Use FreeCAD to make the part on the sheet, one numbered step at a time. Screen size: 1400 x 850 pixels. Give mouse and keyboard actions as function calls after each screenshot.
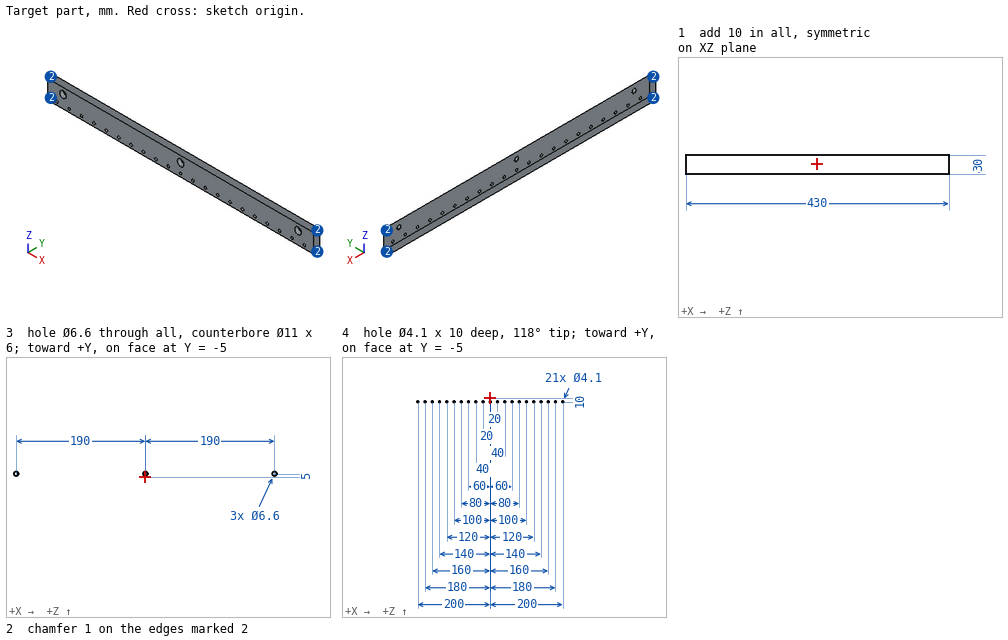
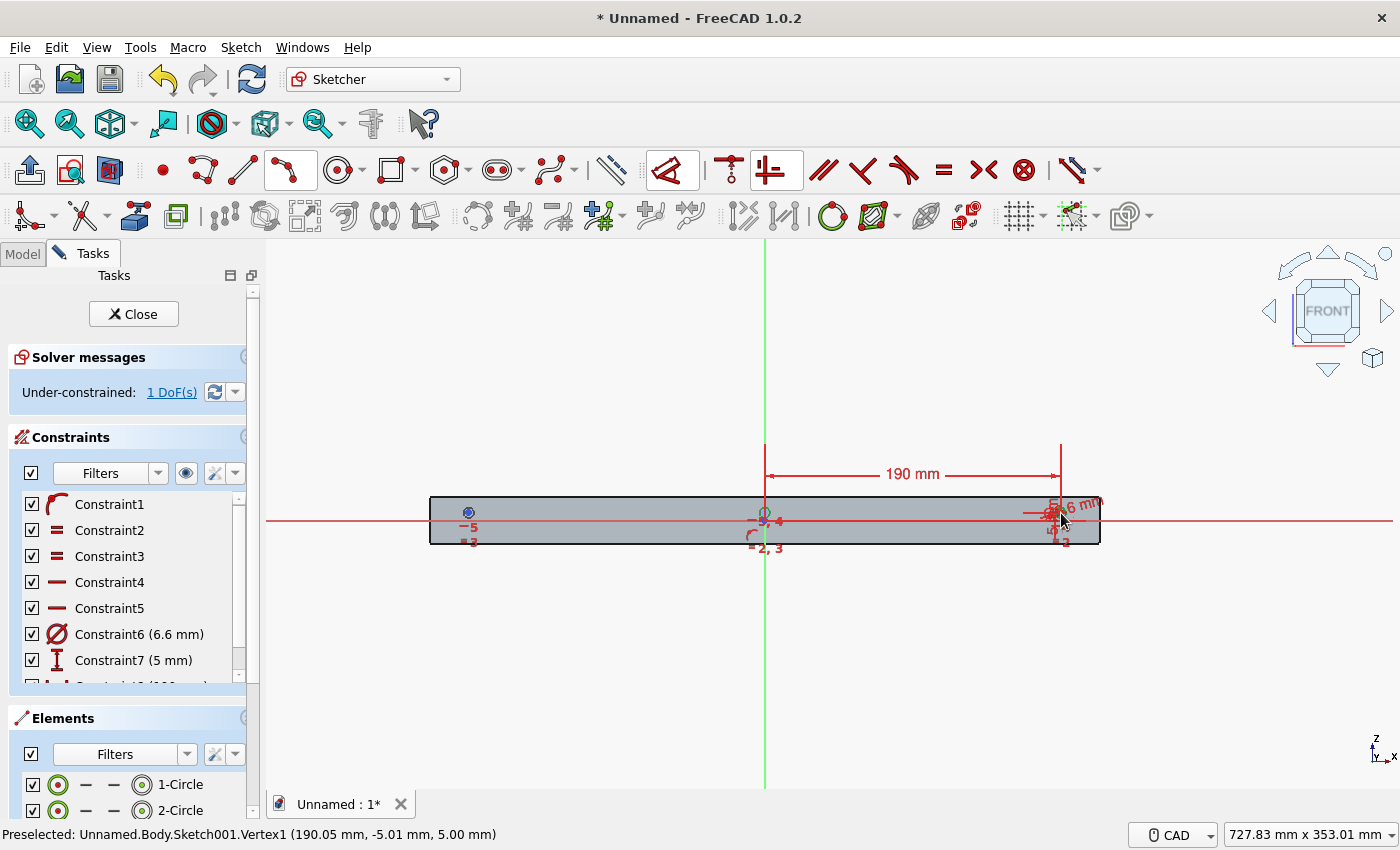
click(469, 513)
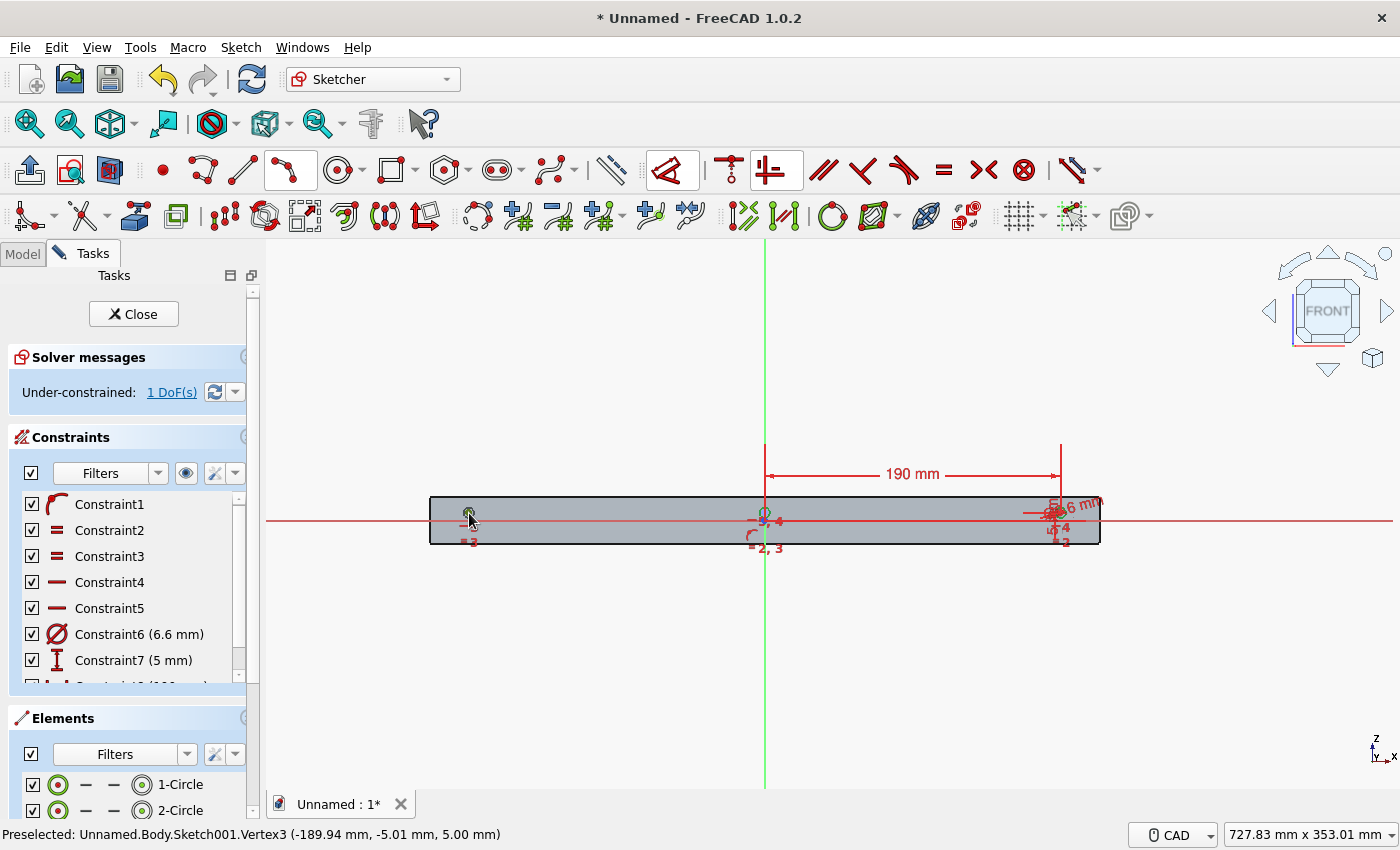
key(l)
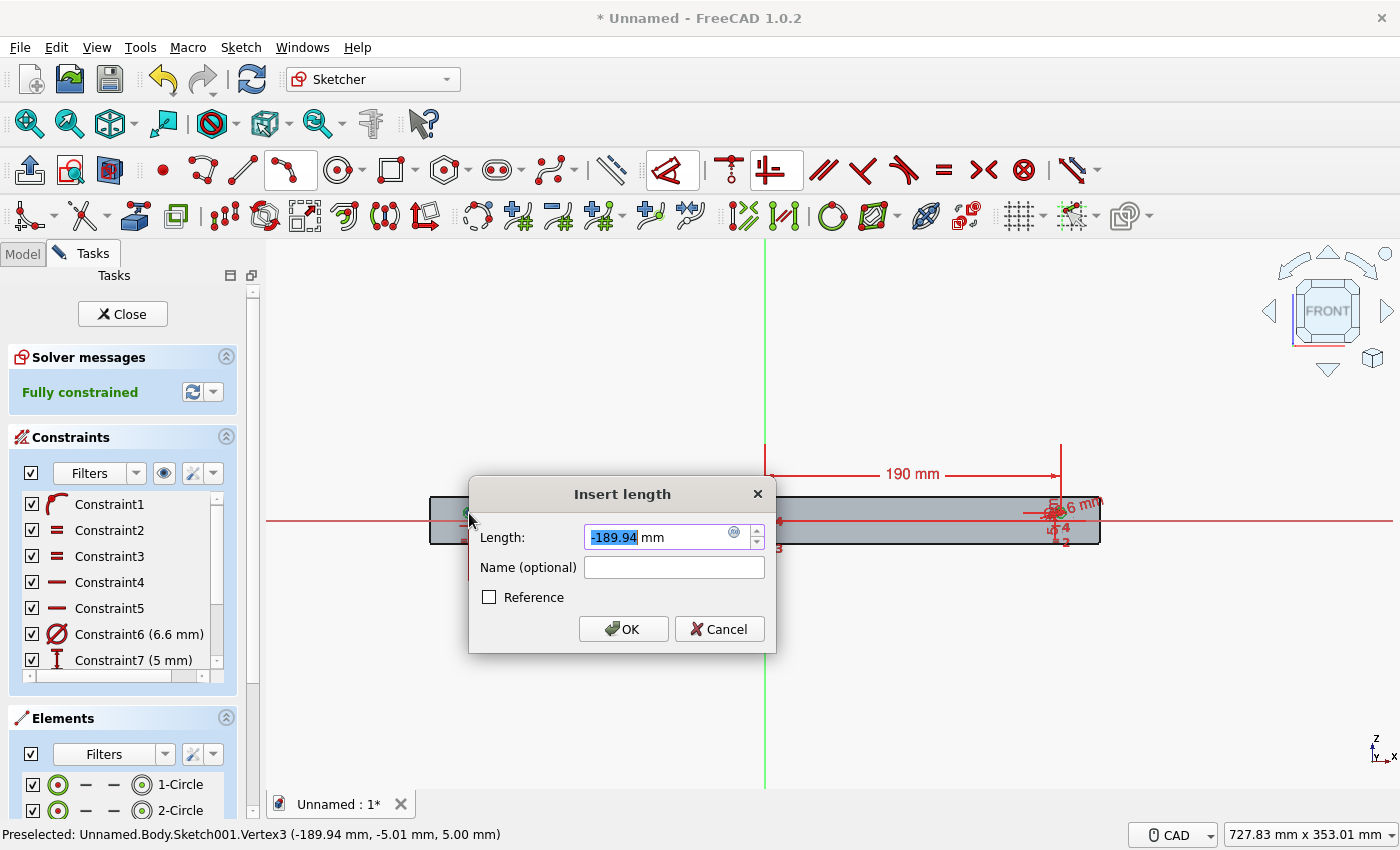
text(-190)
key(Return)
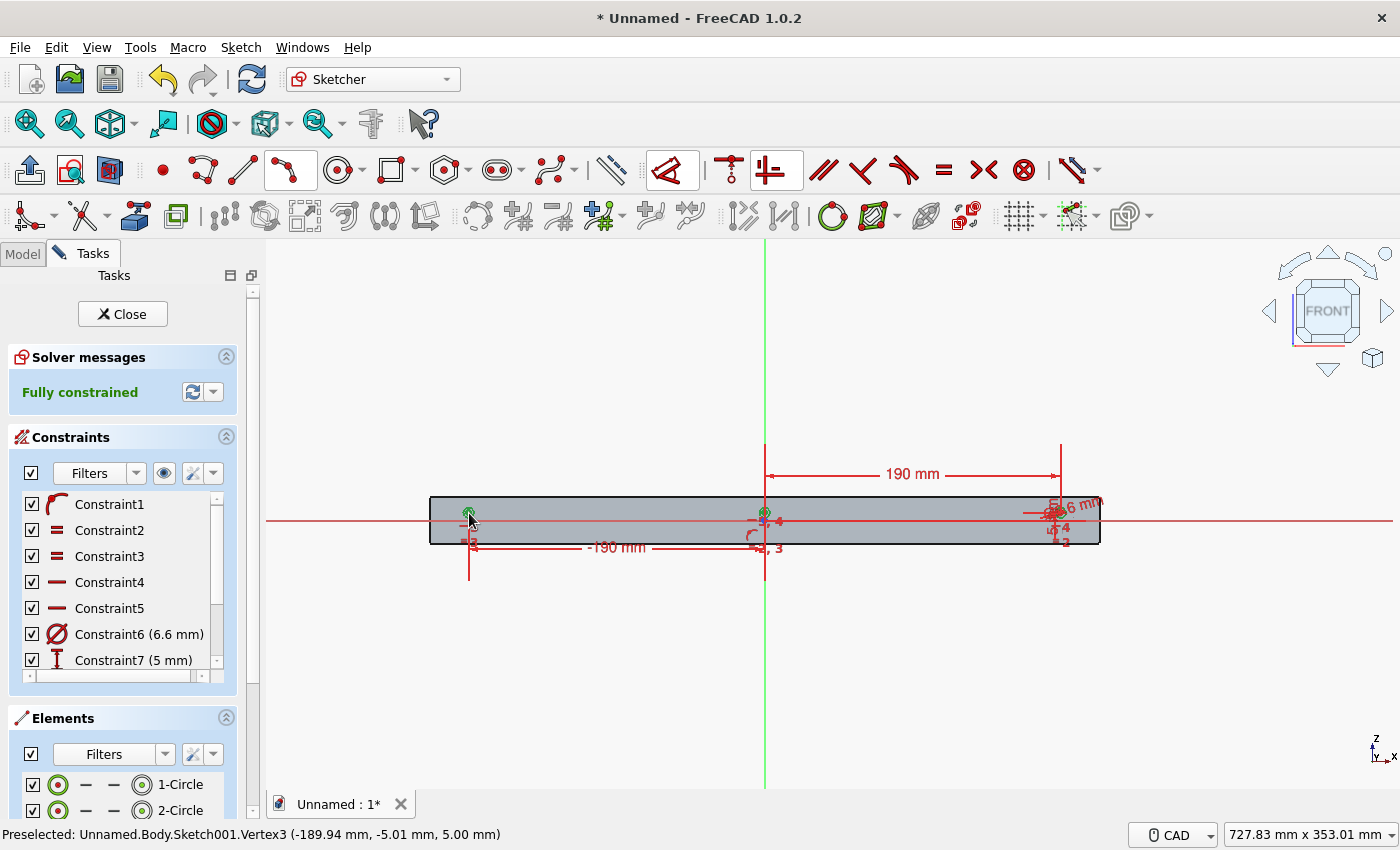
click(123, 314)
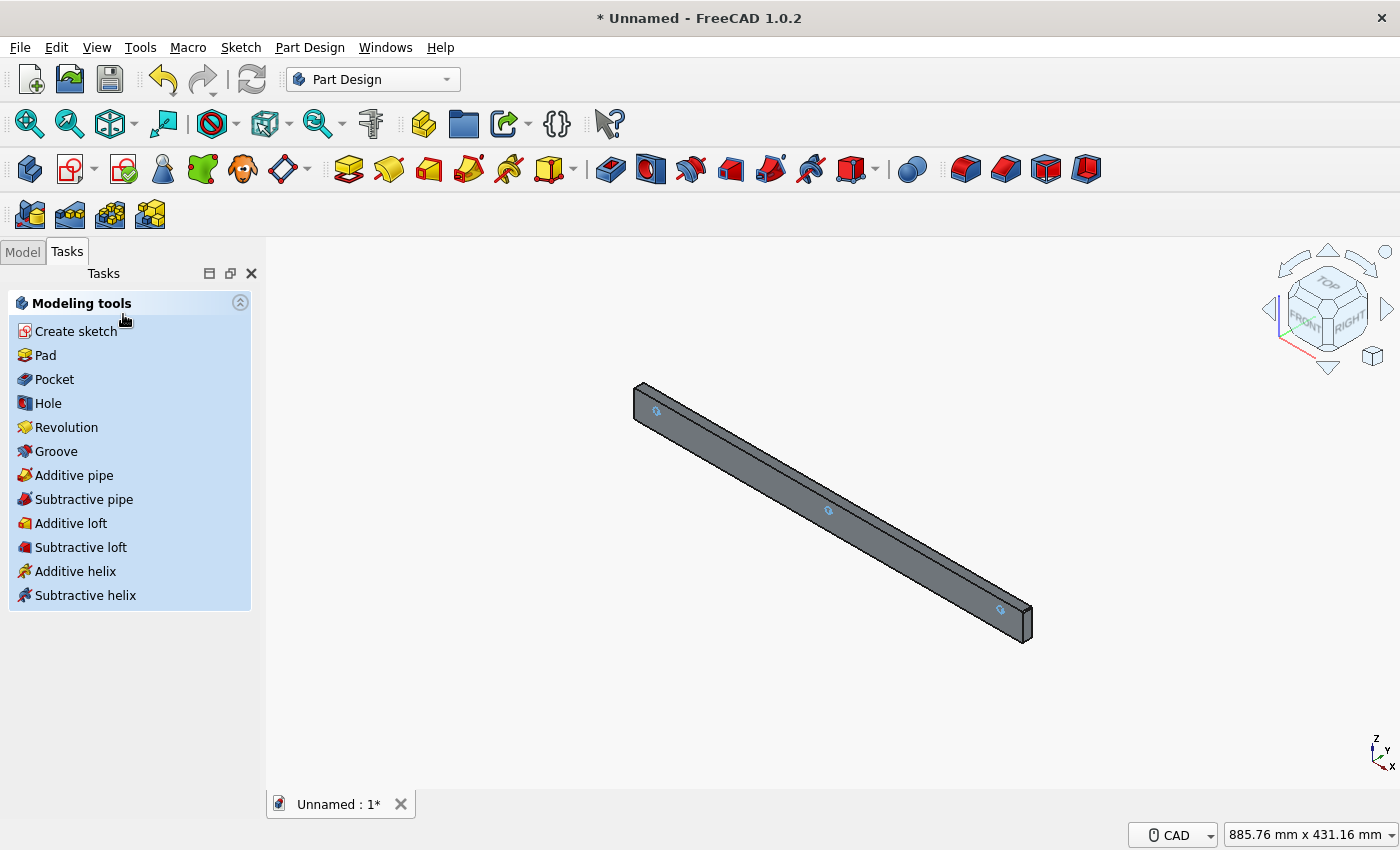
click(652, 170)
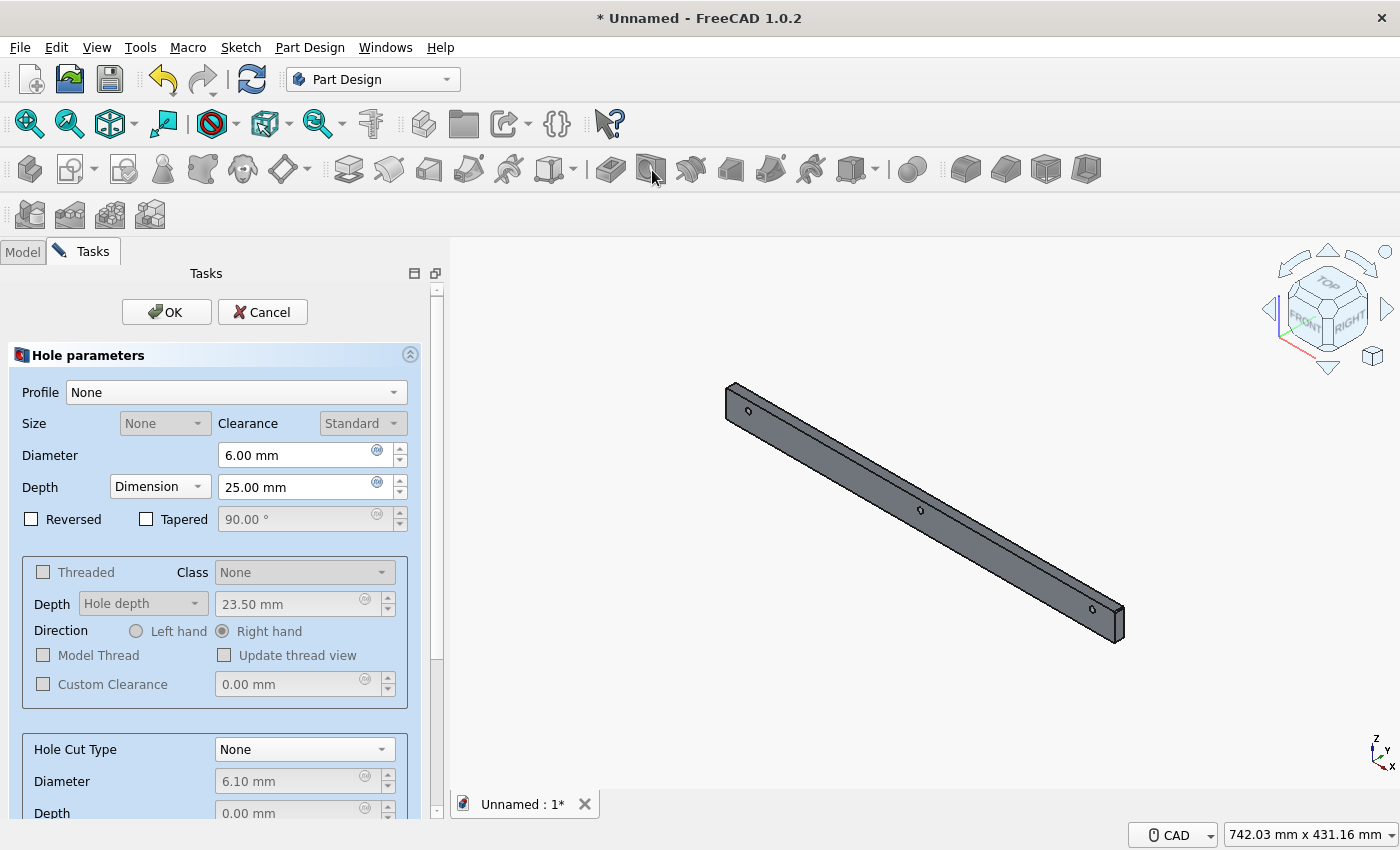
triple_click(305, 455)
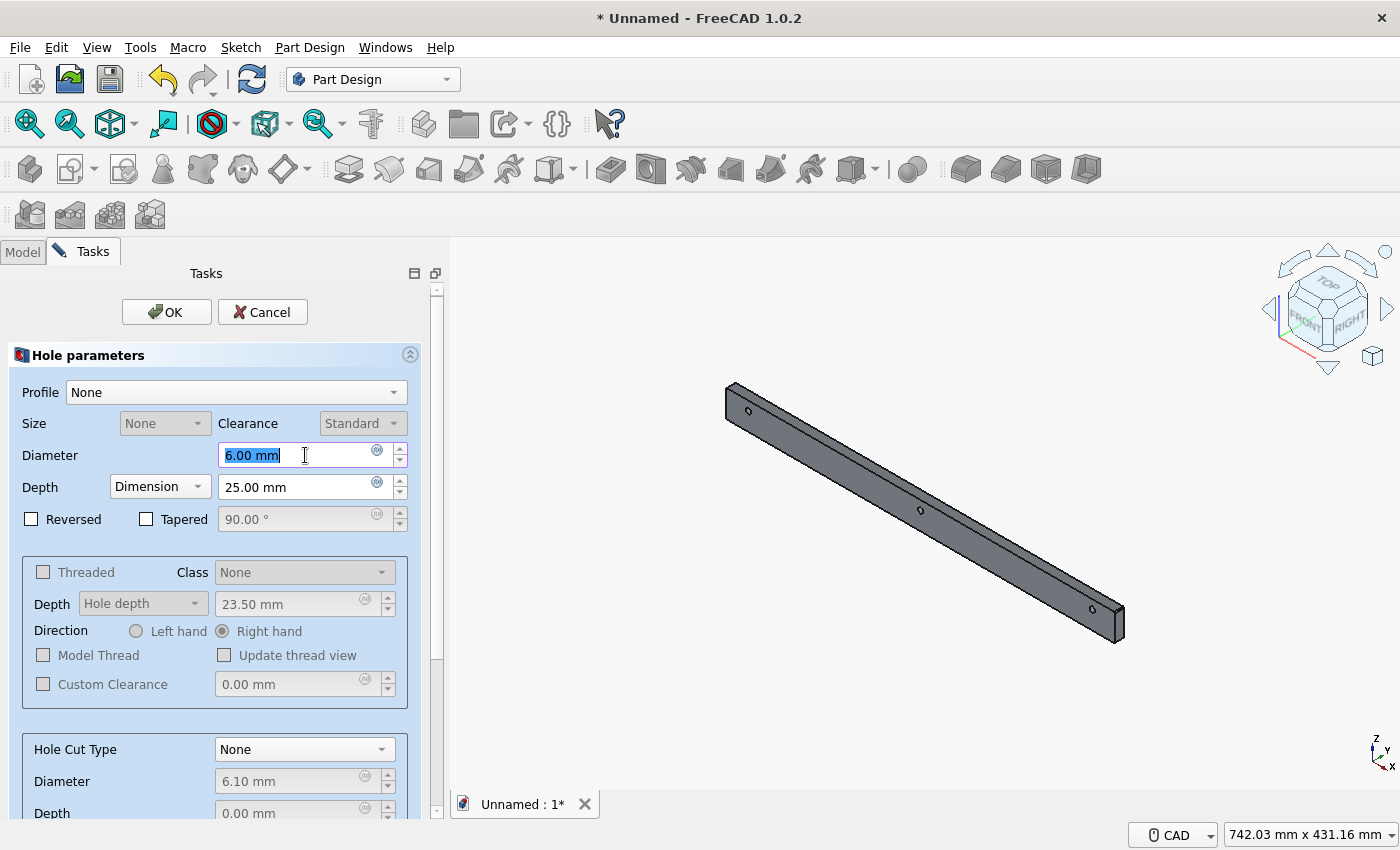
text(6.6)
key(Tab)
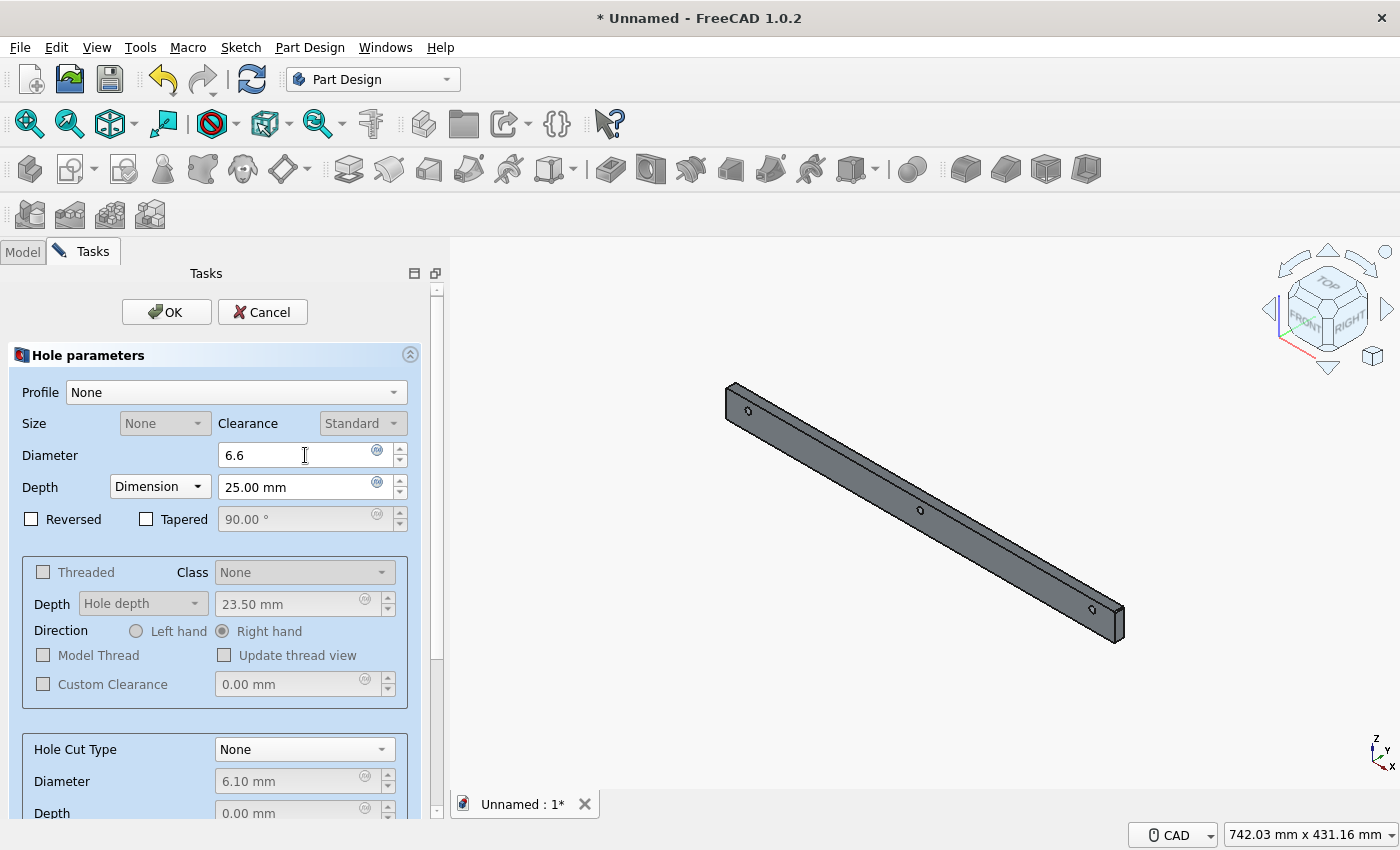
click(161, 486)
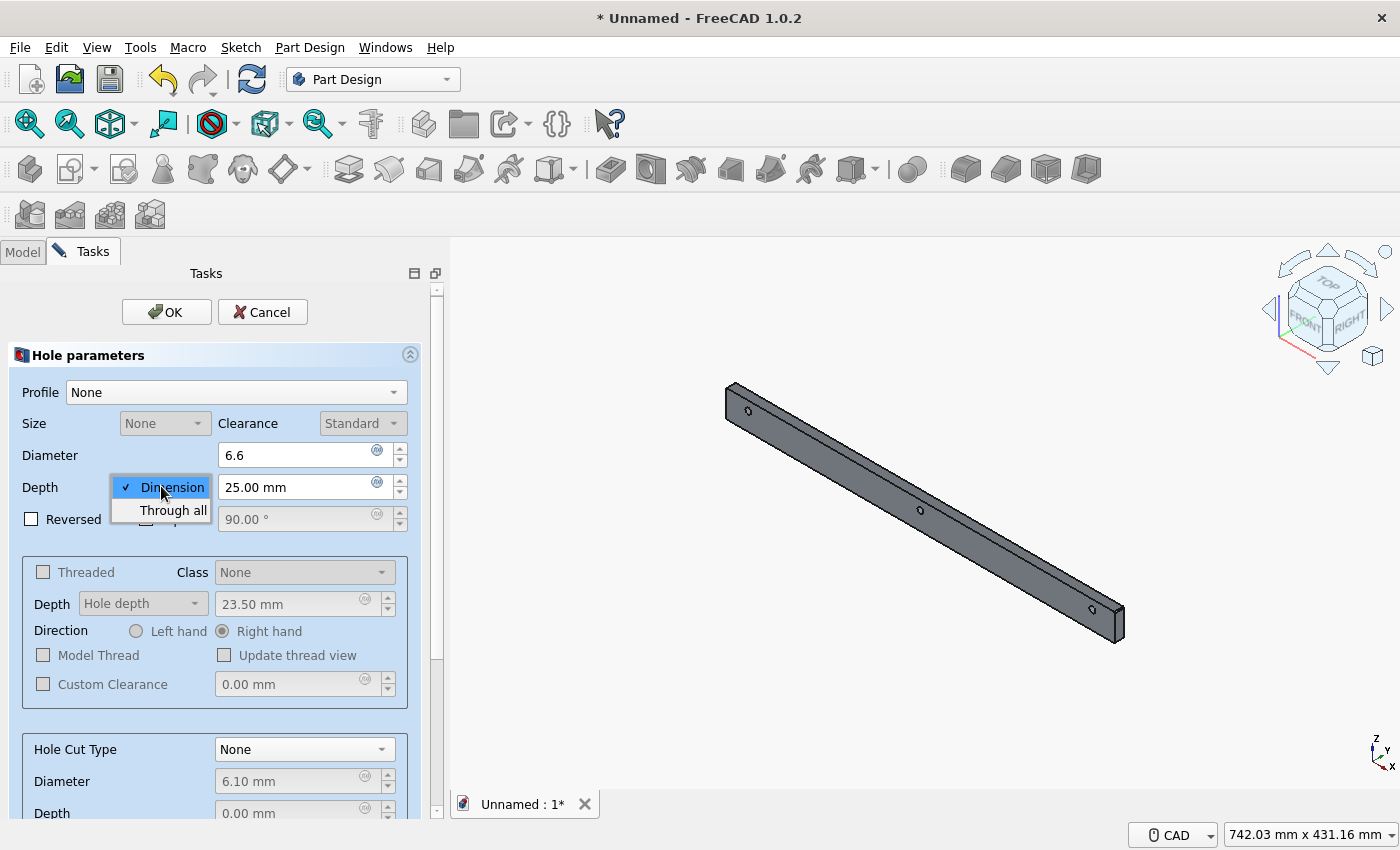
click(160, 510)